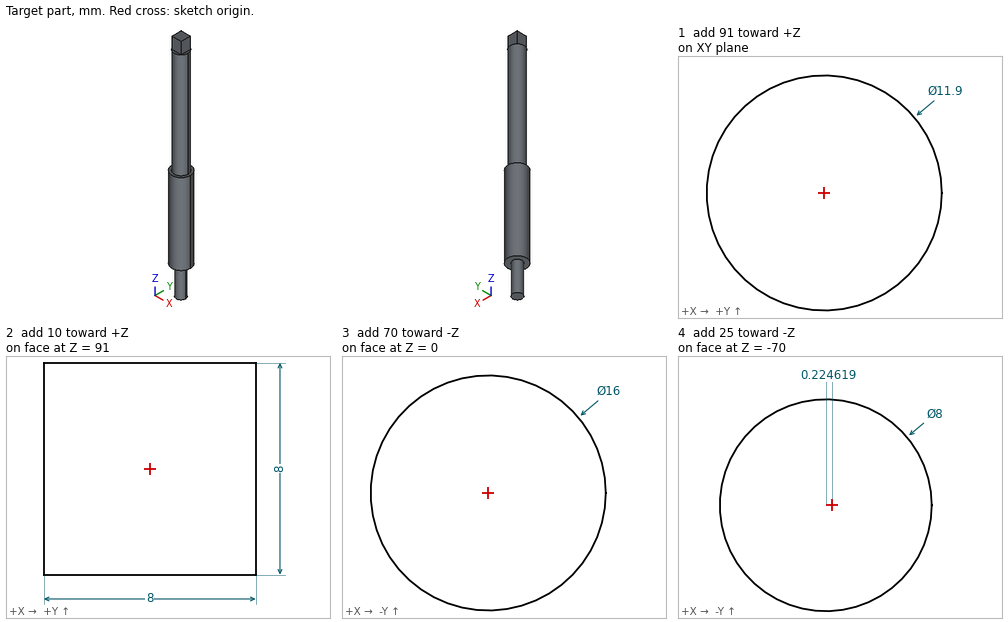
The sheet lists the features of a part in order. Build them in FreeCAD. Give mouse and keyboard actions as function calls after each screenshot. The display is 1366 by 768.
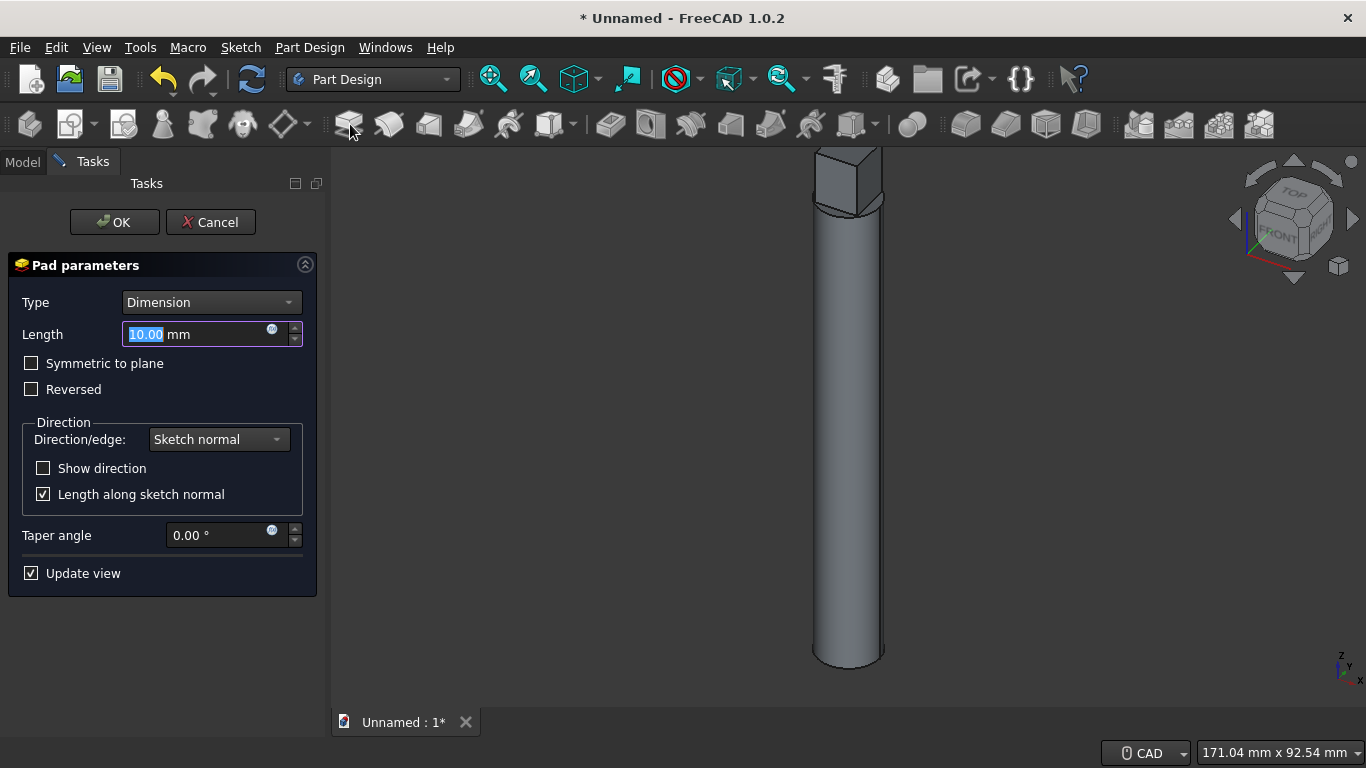
text(10)
key(Tab)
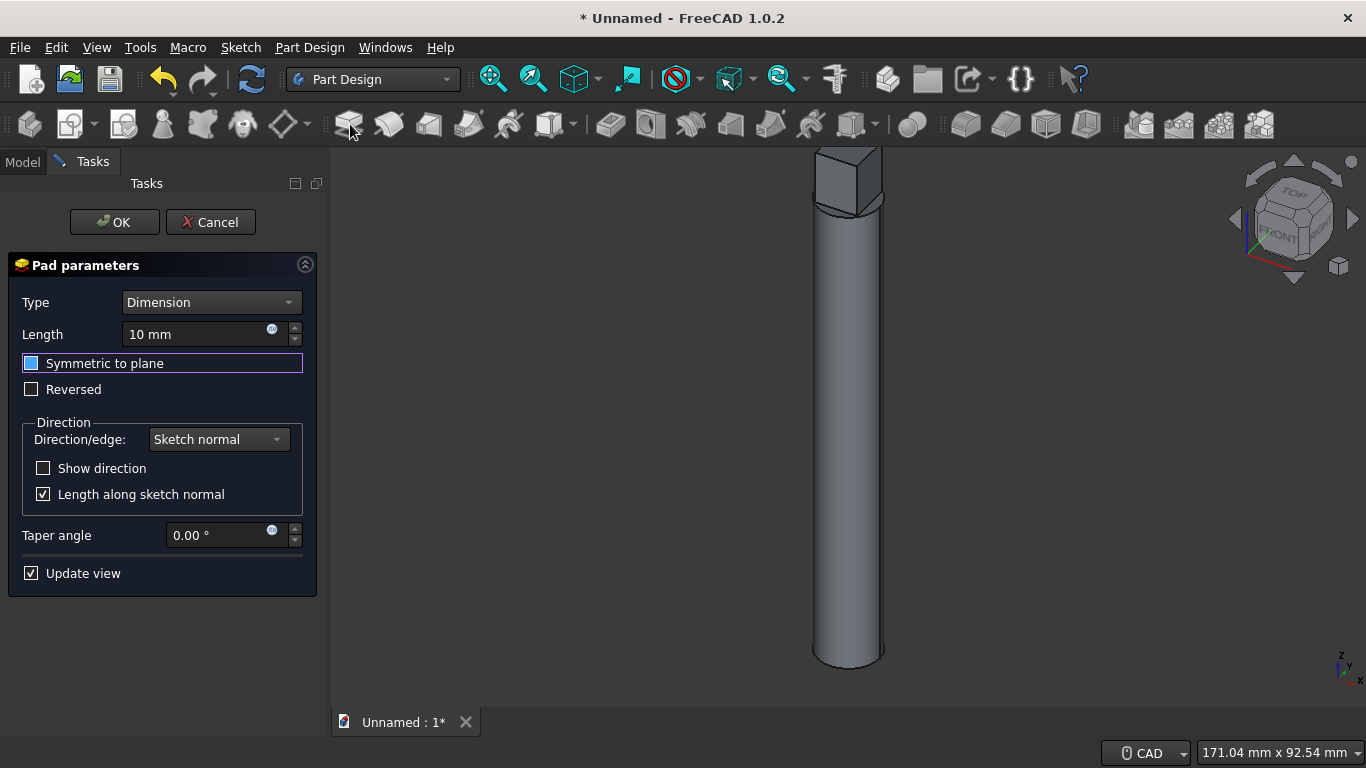
click(115, 222)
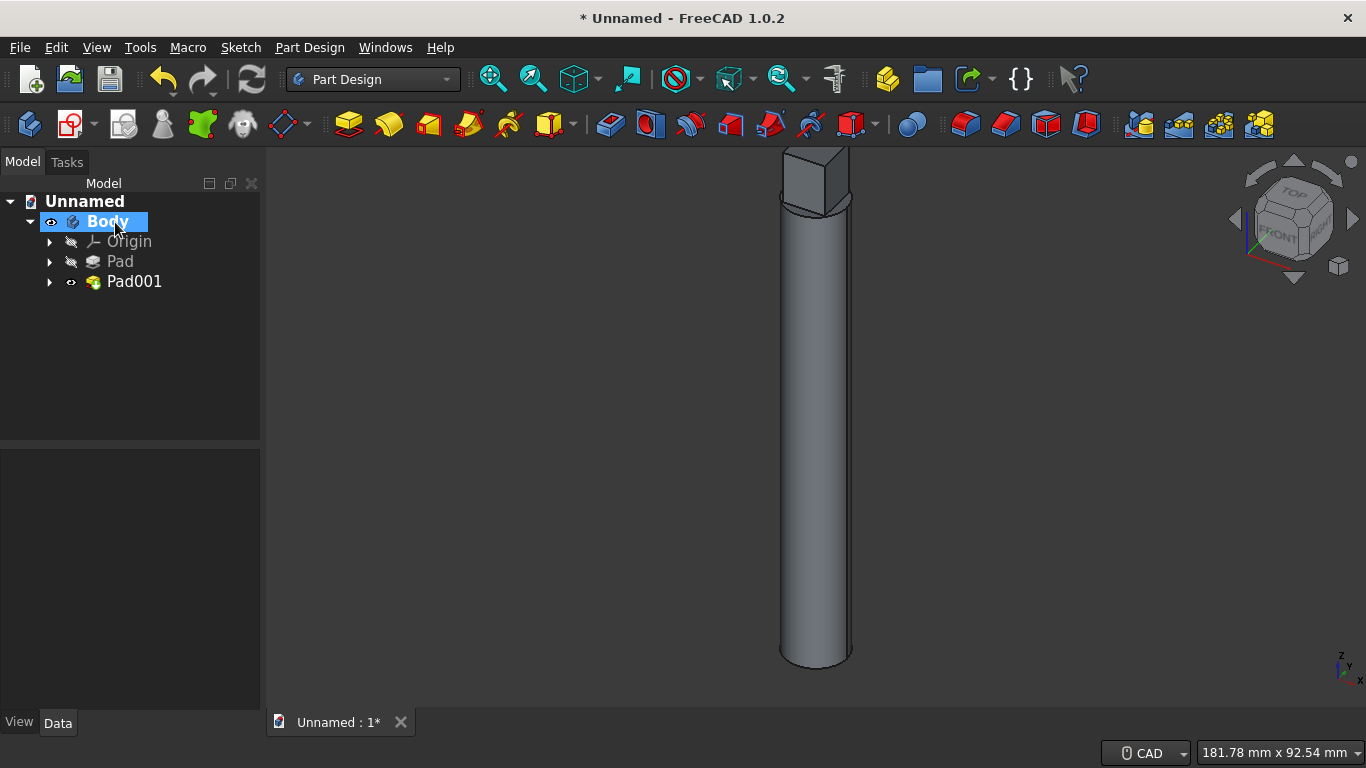
click(494, 80)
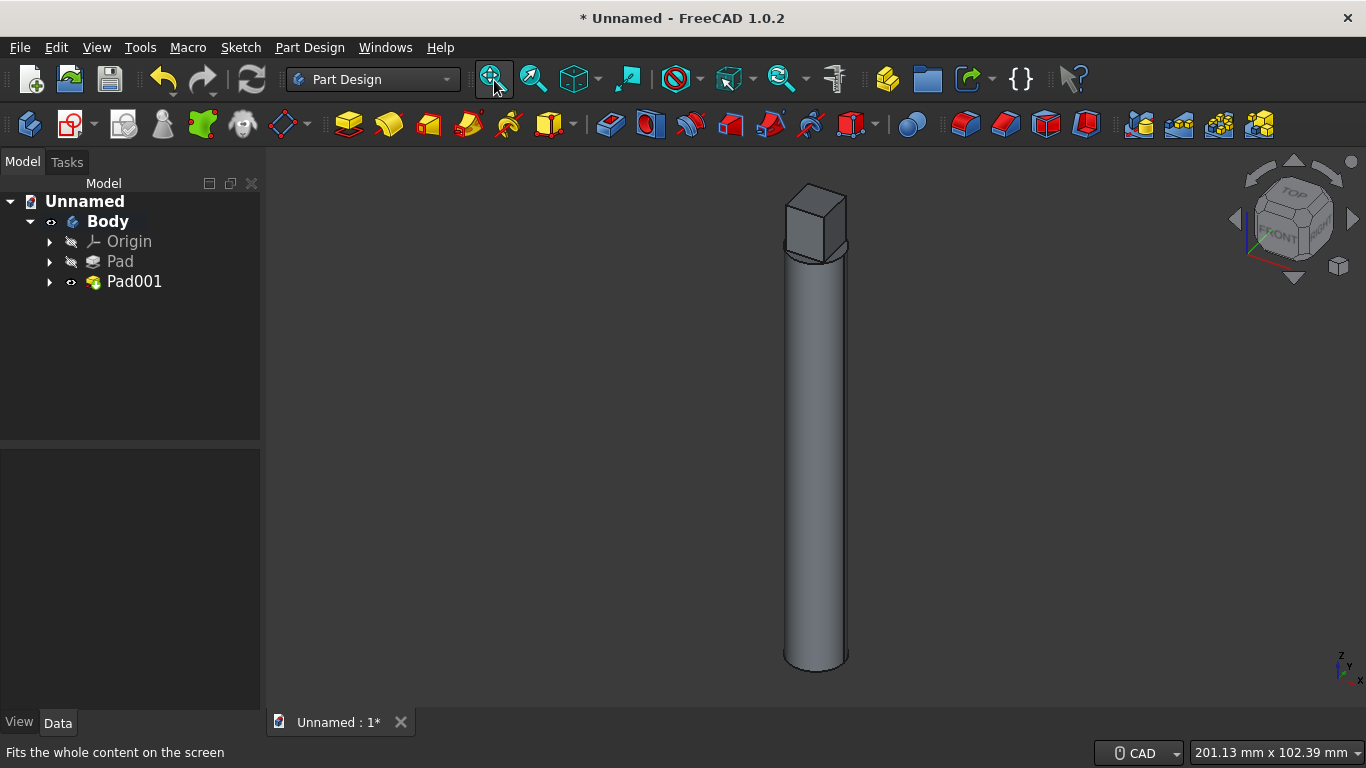
key(5)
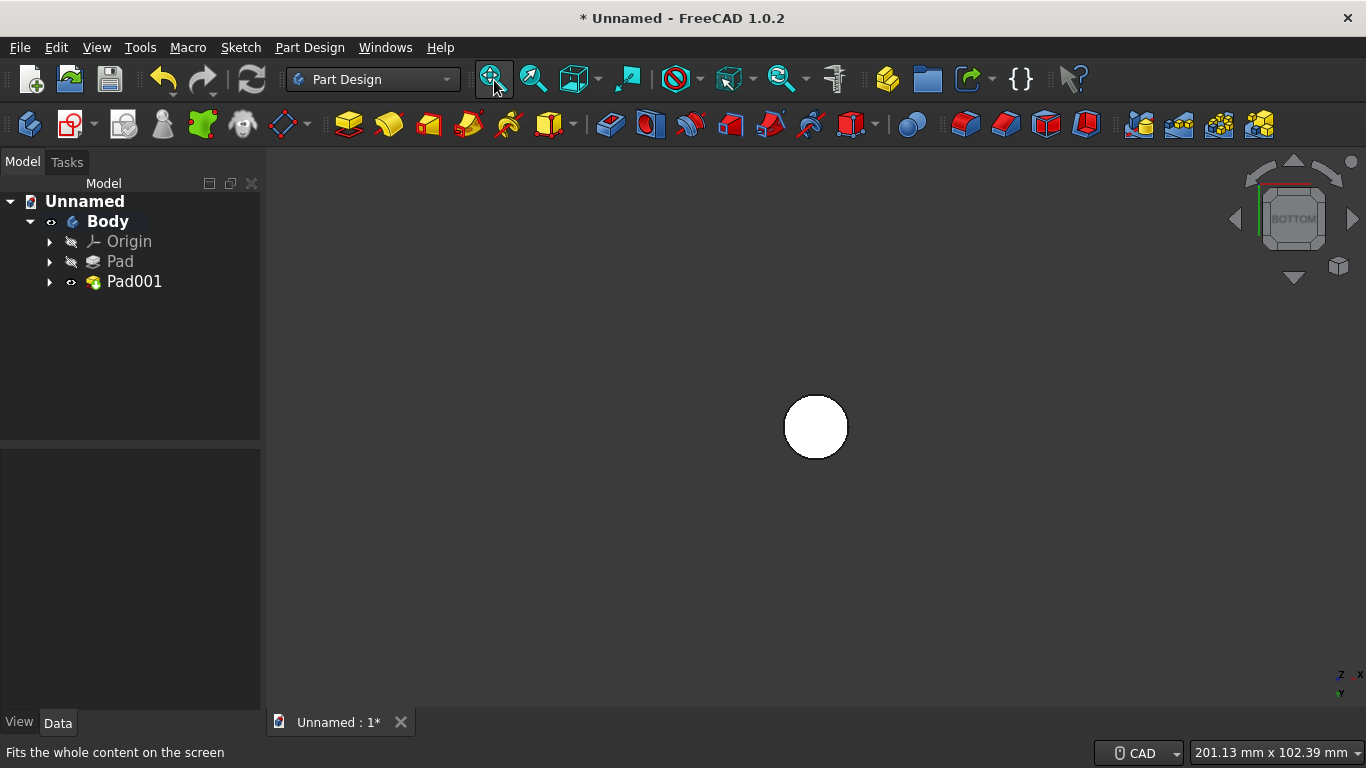
key(v)
key(f)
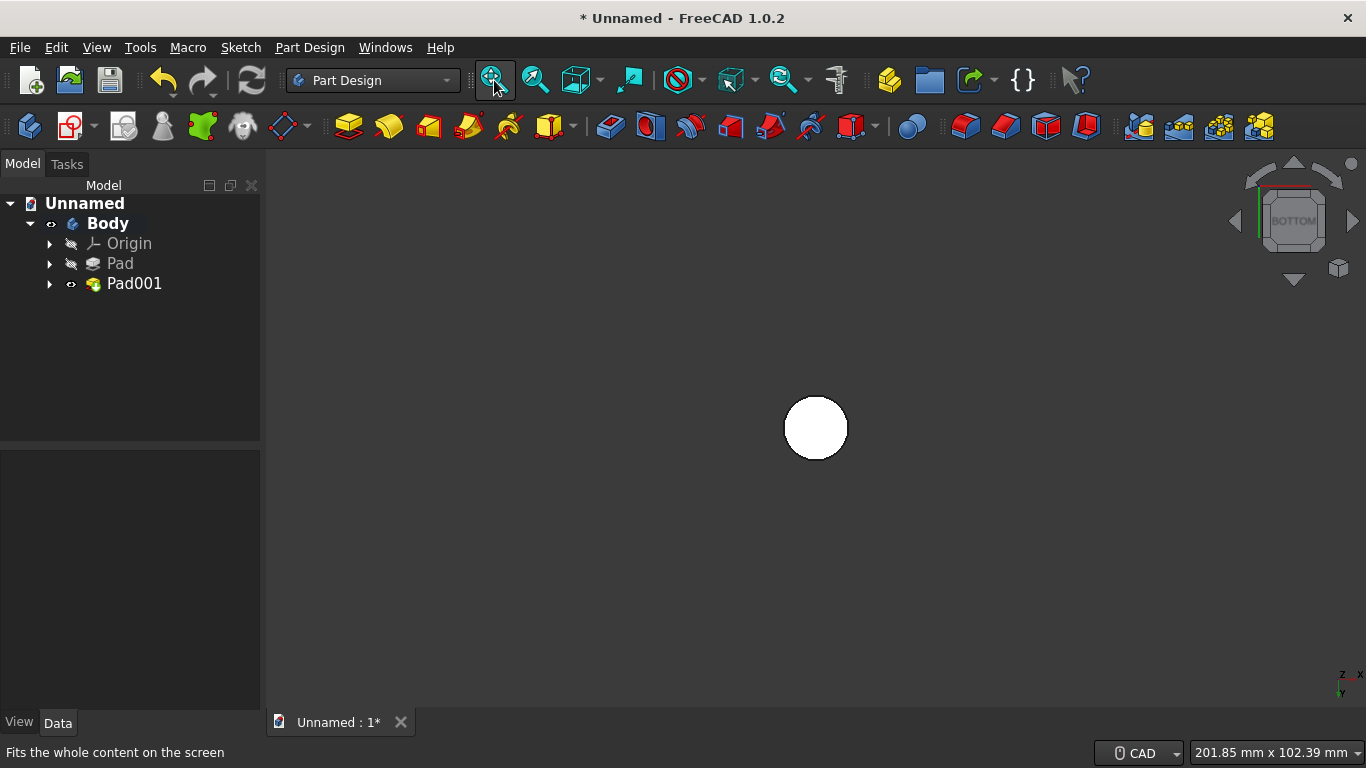
click(816, 427)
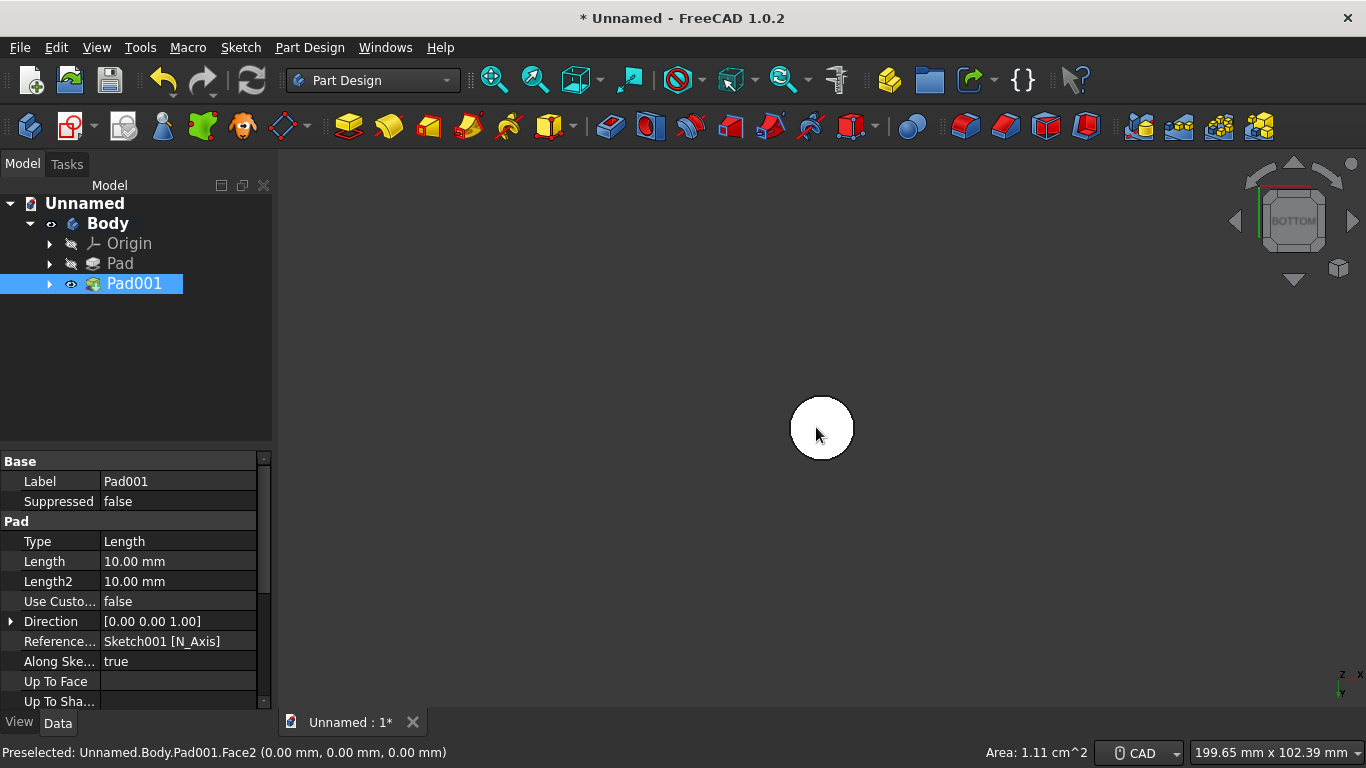
click(70, 126)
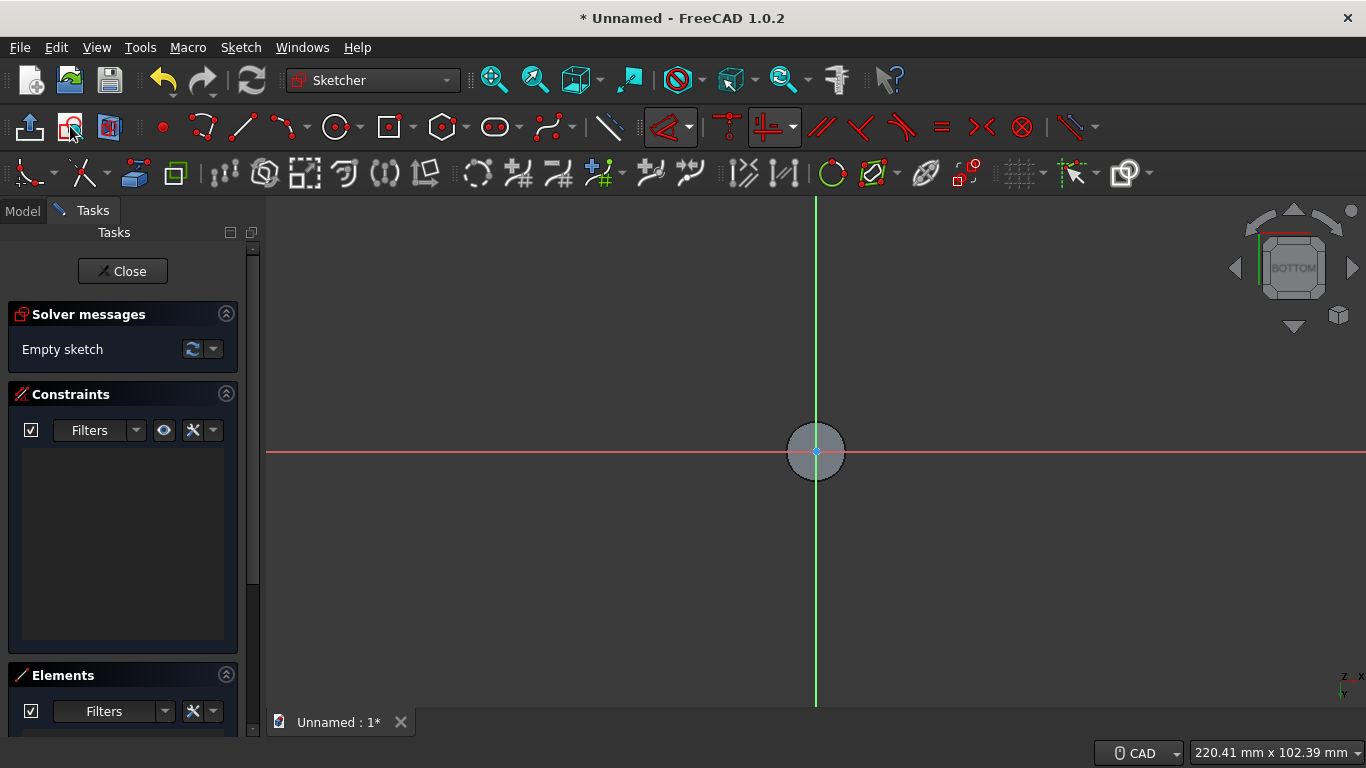
scroll(838, 452, up, 7)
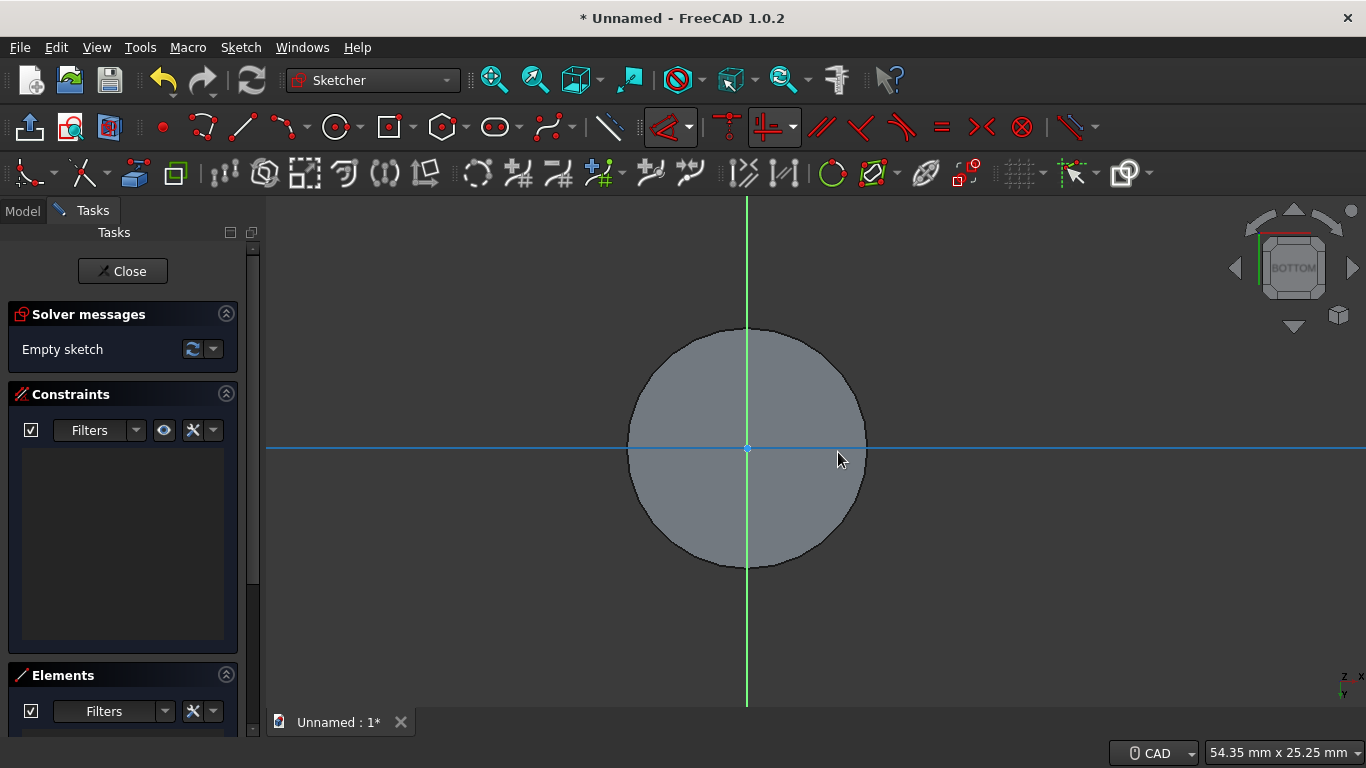
click(336, 128)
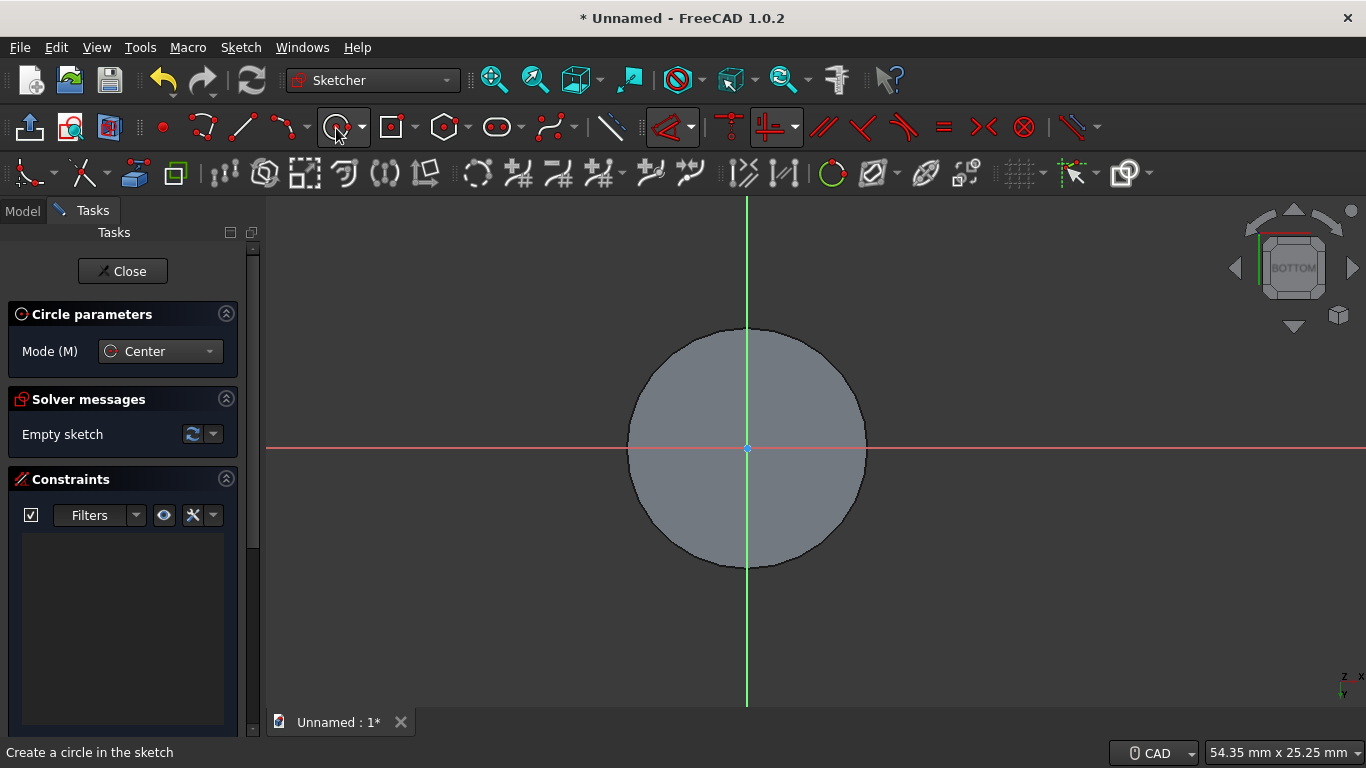
click(747, 448)
click(862, 334)
key(Escape)